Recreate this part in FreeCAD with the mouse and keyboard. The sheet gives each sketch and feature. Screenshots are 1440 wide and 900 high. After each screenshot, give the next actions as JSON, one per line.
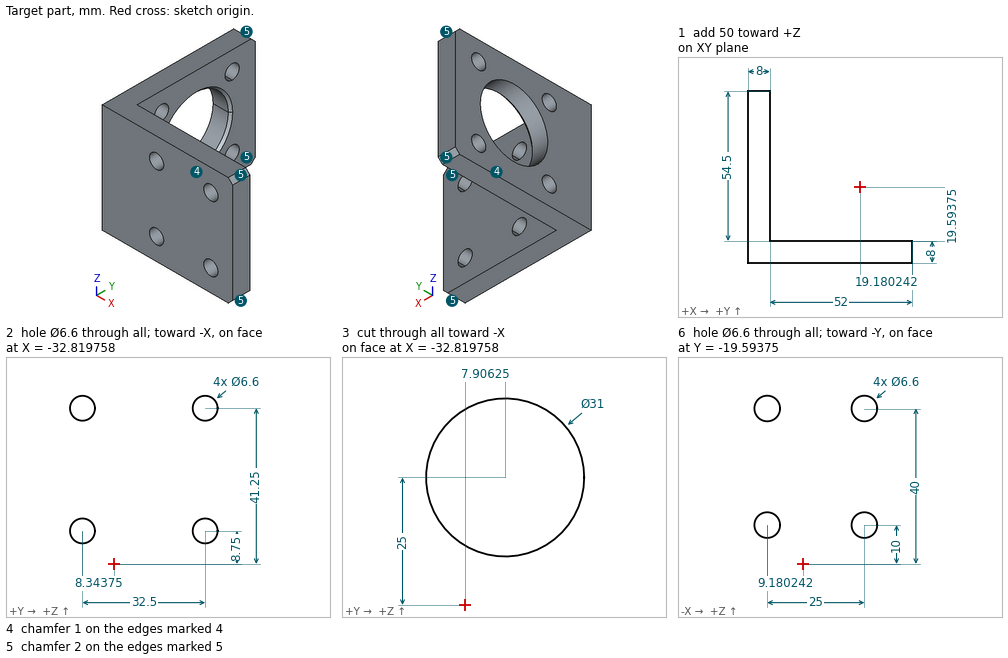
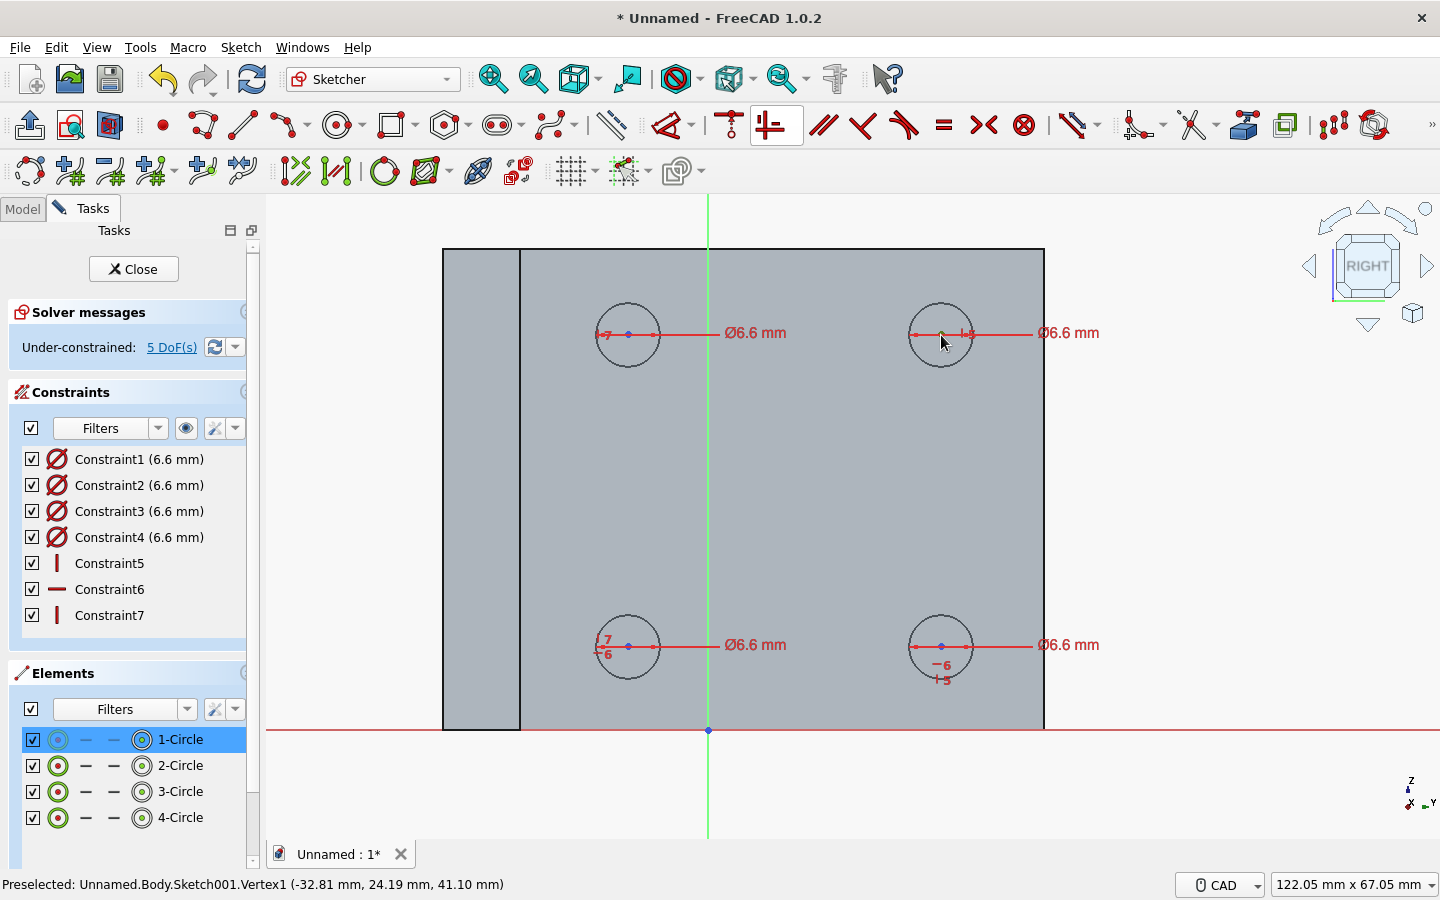
{"action": "left_click", "coordinate": [628, 335]}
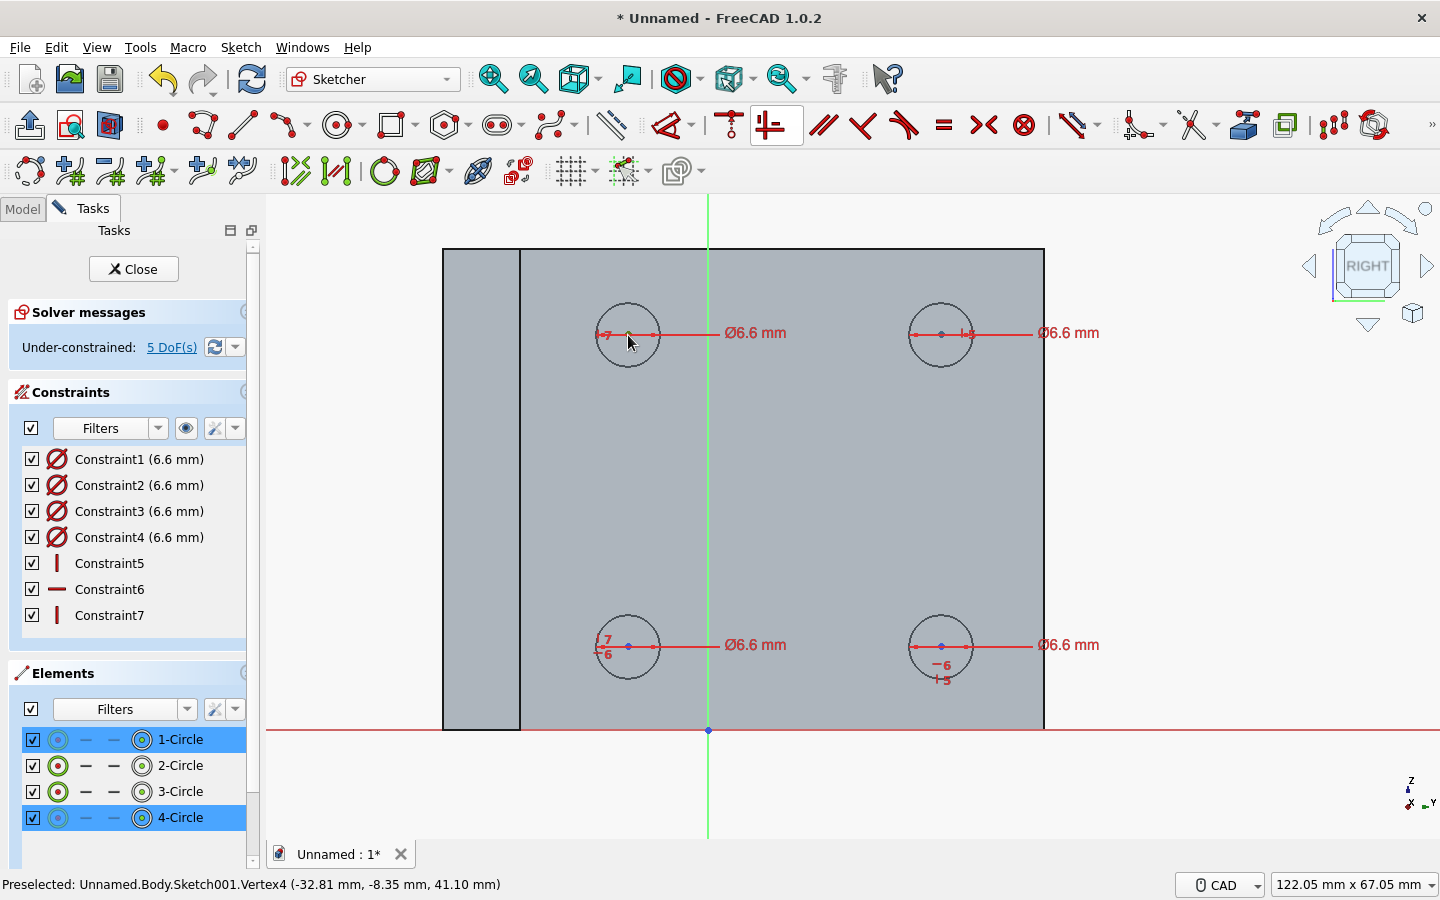
{"action": "left_click", "coordinate": [798, 126]}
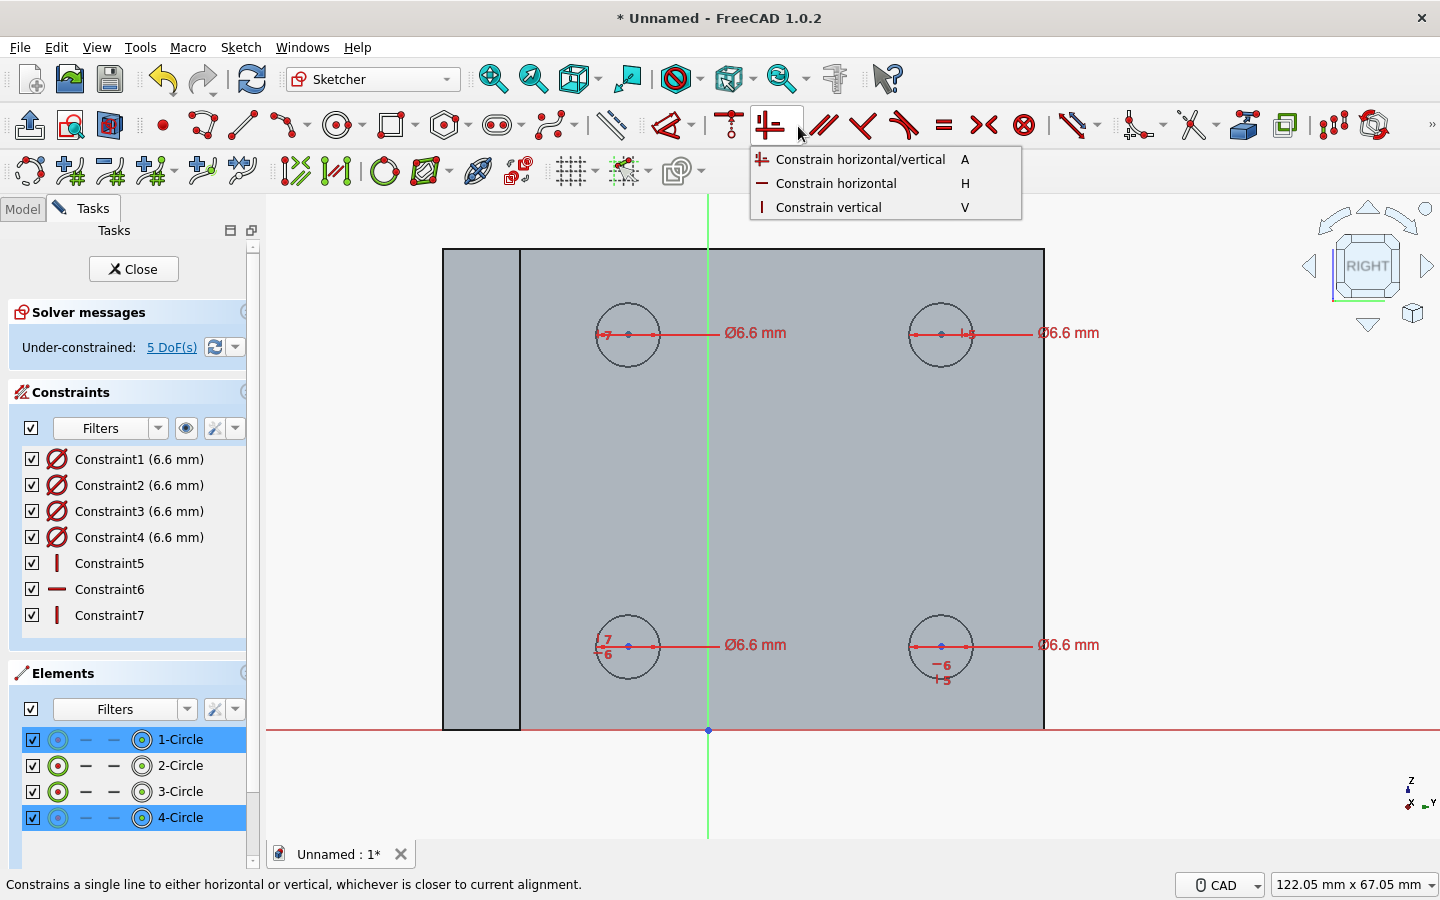
{"action": "left_click", "coordinate": [886, 183]}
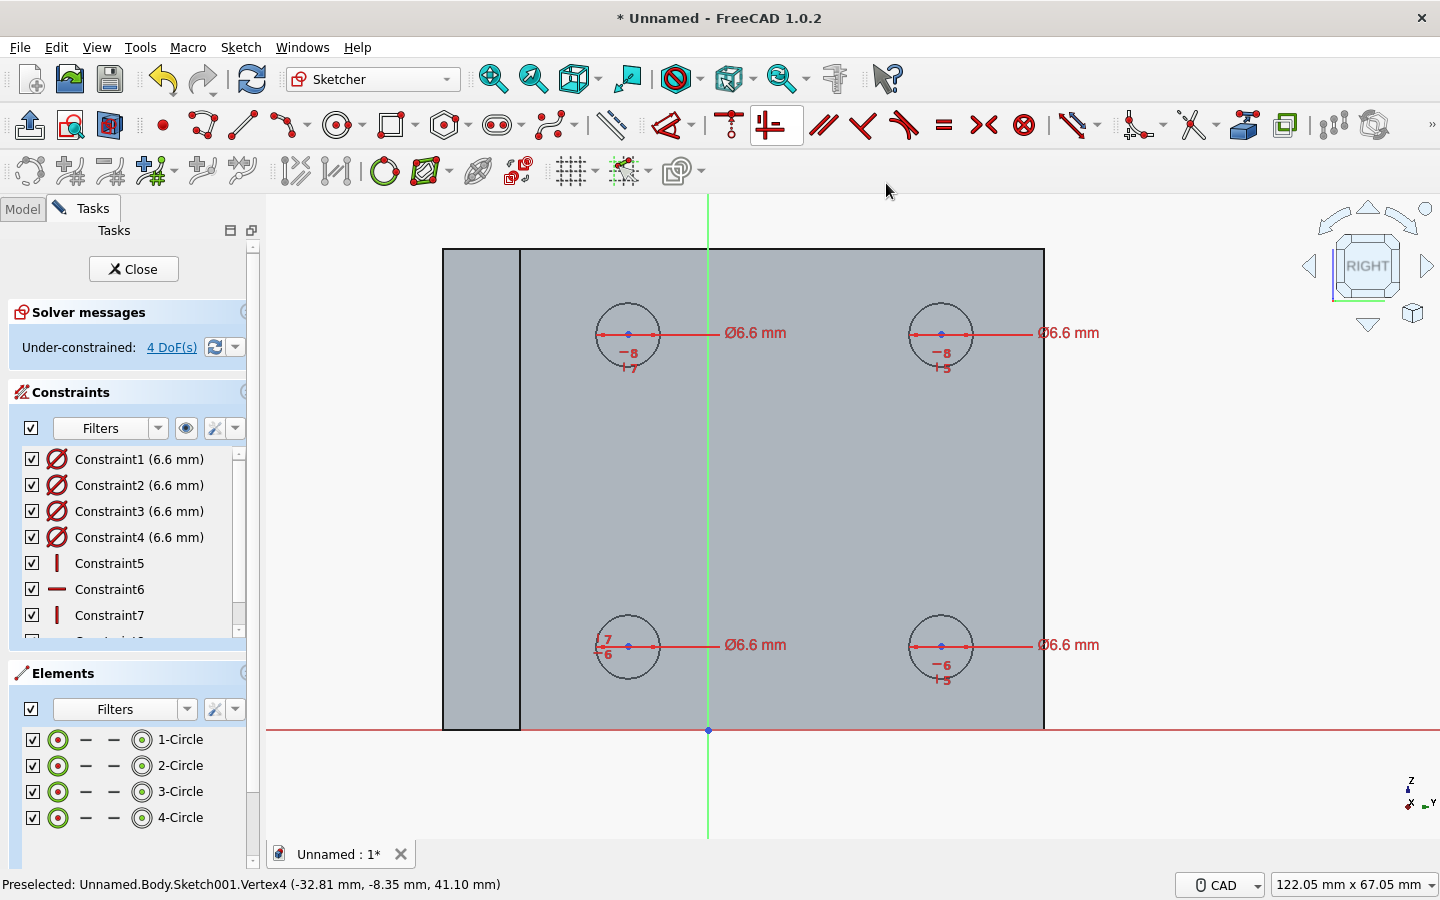
{"action": "key", "text": "d"}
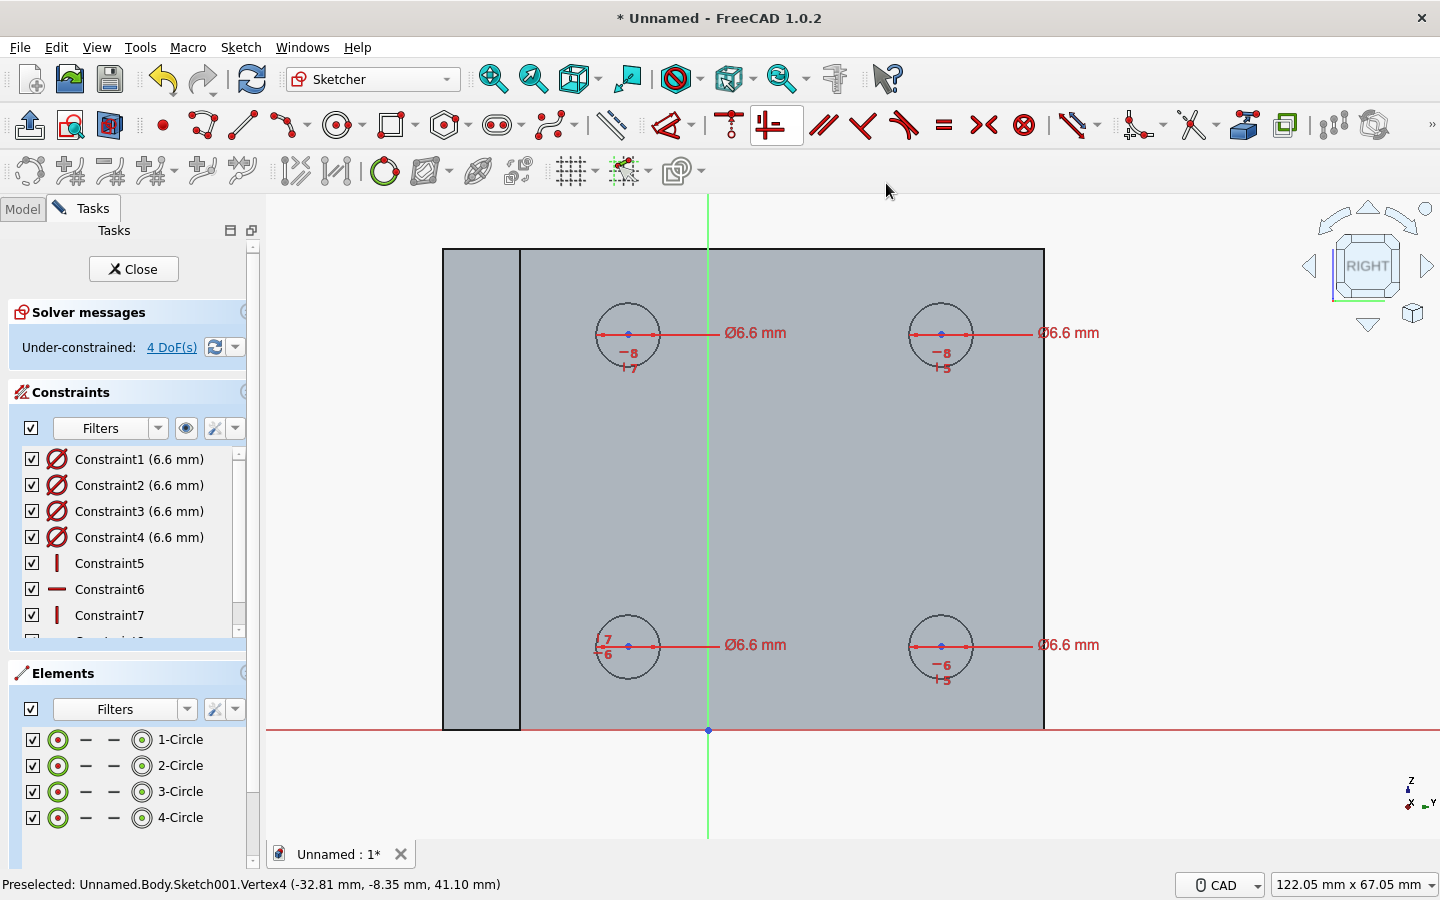
{"action": "left_click", "coordinate": [941, 647]}
{"action": "left_click", "coordinate": [975, 689]}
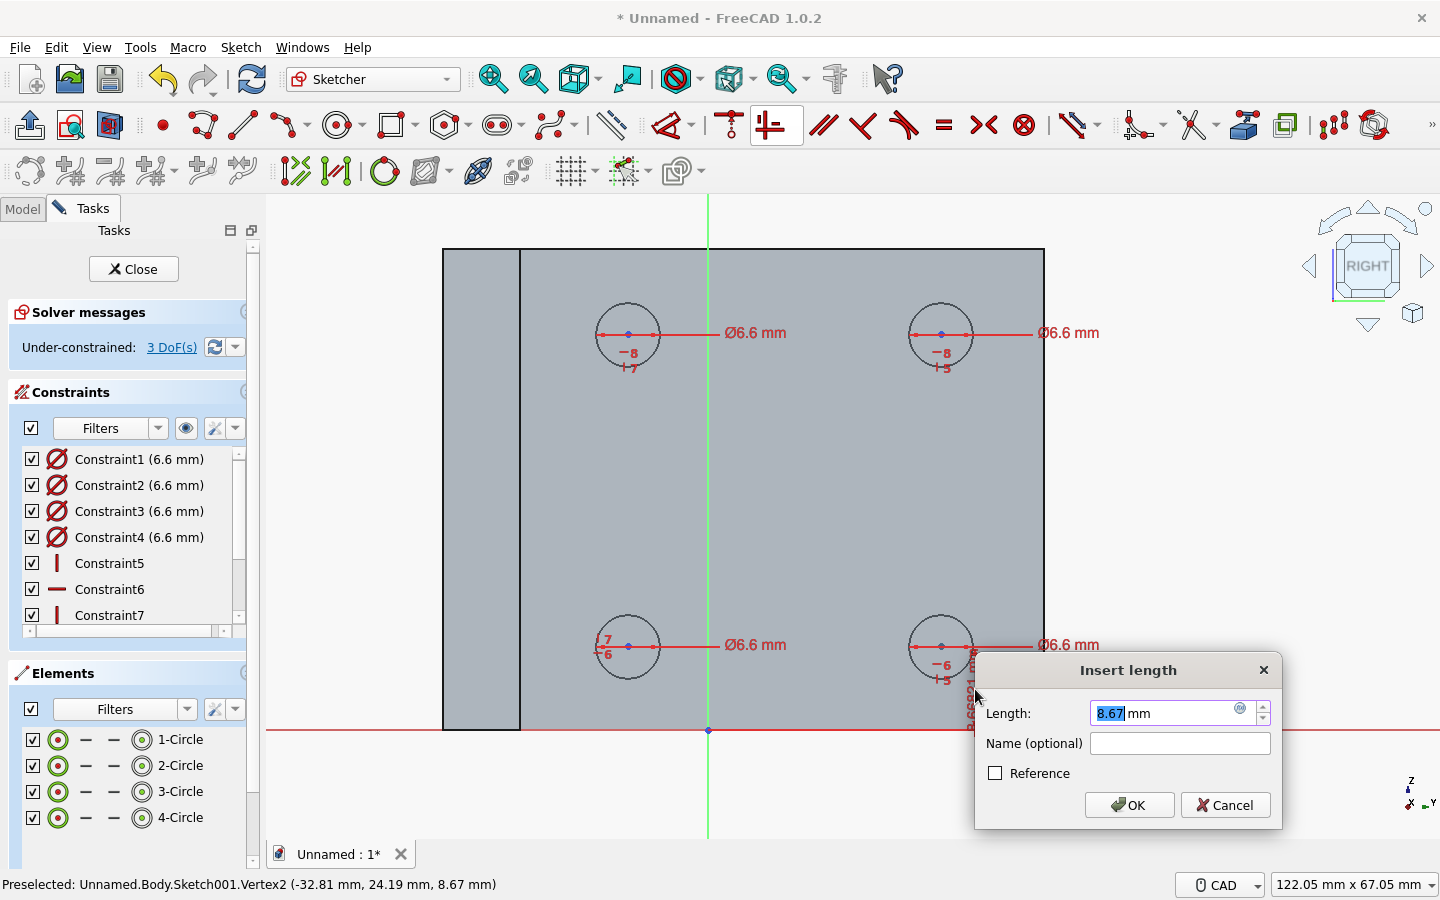
{"action": "type", "text": "8.75"}
{"action": "key", "text": "Return"}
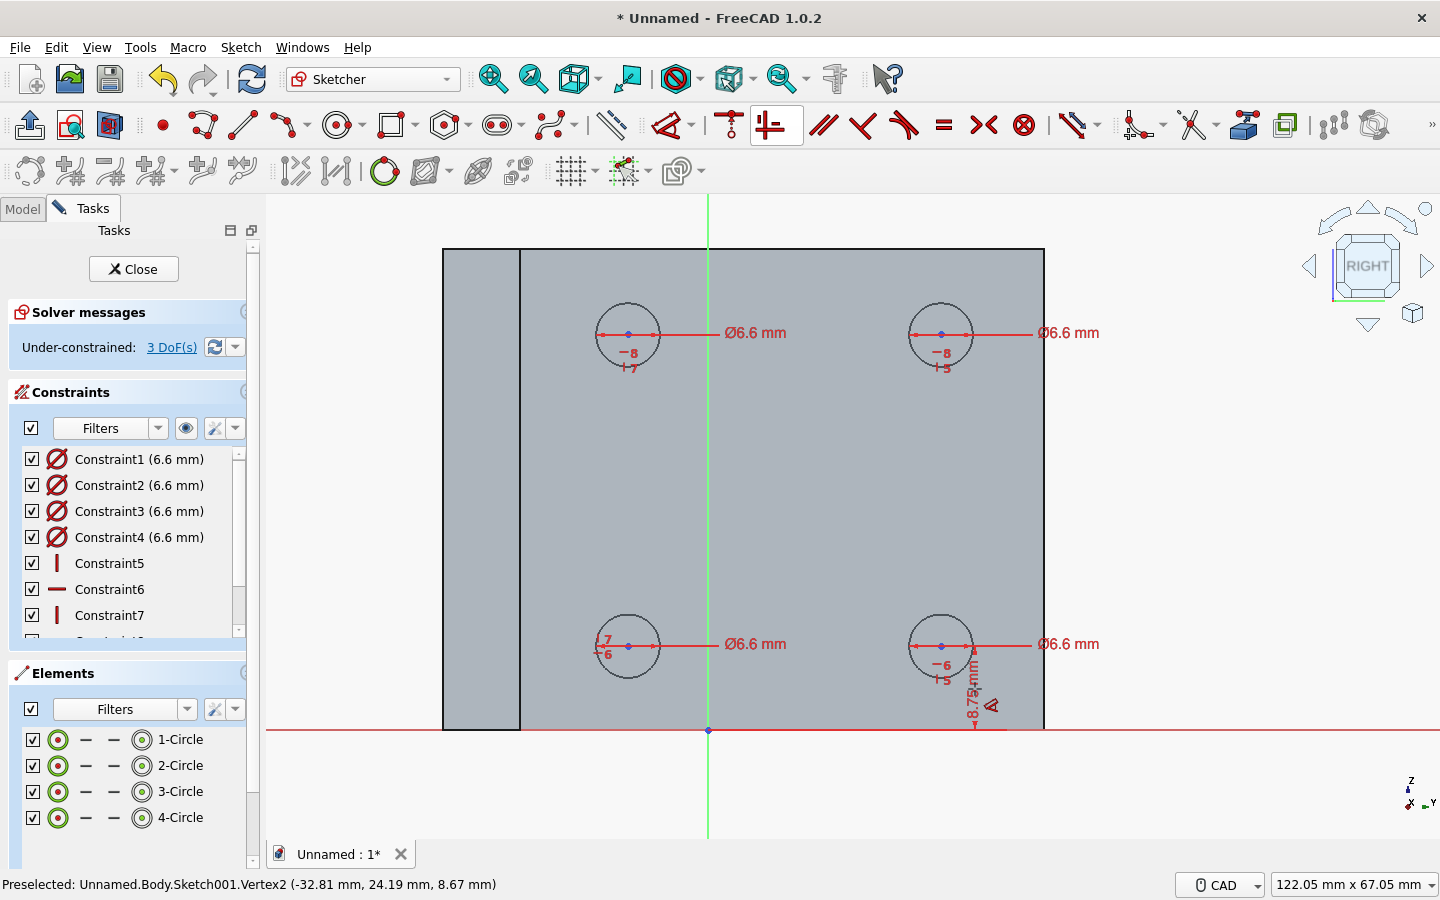
{"action": "left_click", "coordinate": [941, 335]}
{"action": "left_click", "coordinate": [975, 533]}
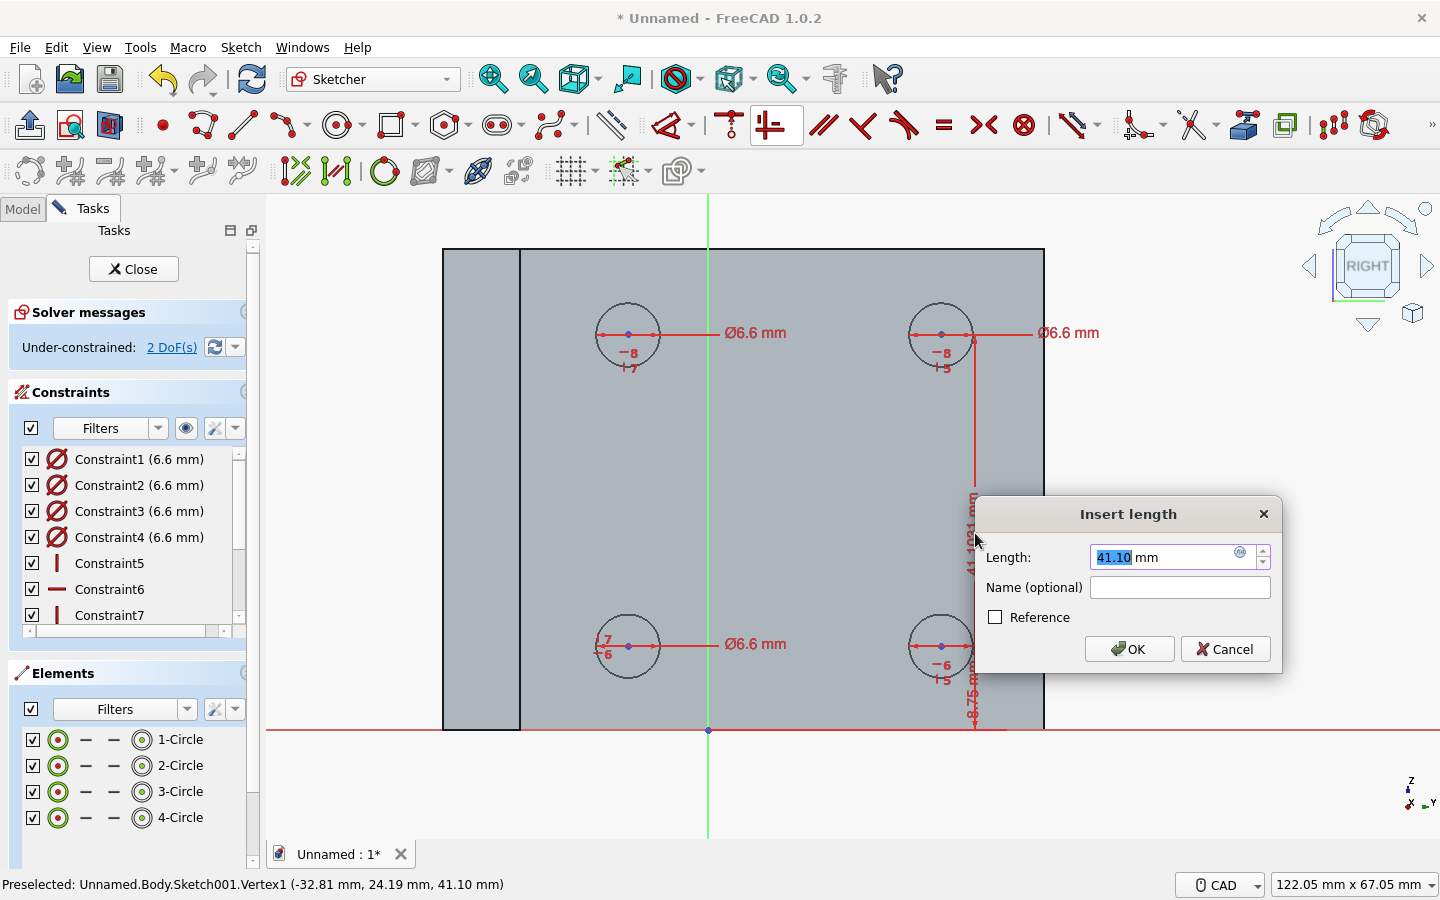
{"action": "type", "text": "41.25"}
{"action": "key", "text": "Return"}